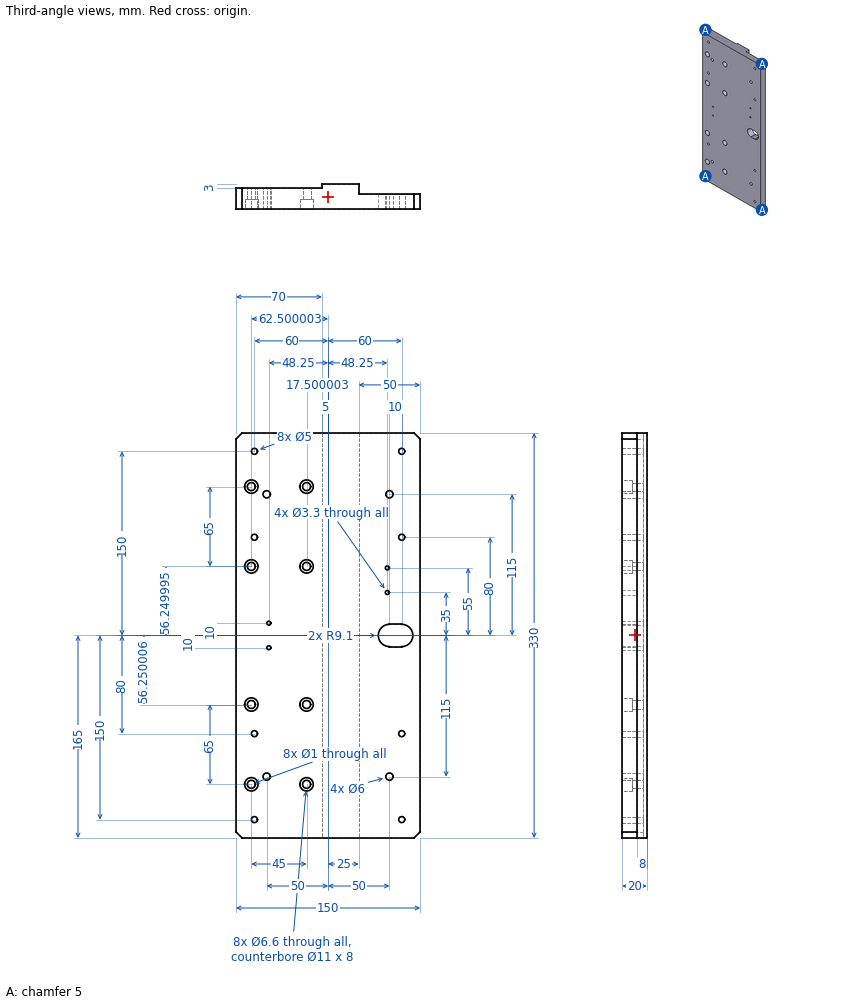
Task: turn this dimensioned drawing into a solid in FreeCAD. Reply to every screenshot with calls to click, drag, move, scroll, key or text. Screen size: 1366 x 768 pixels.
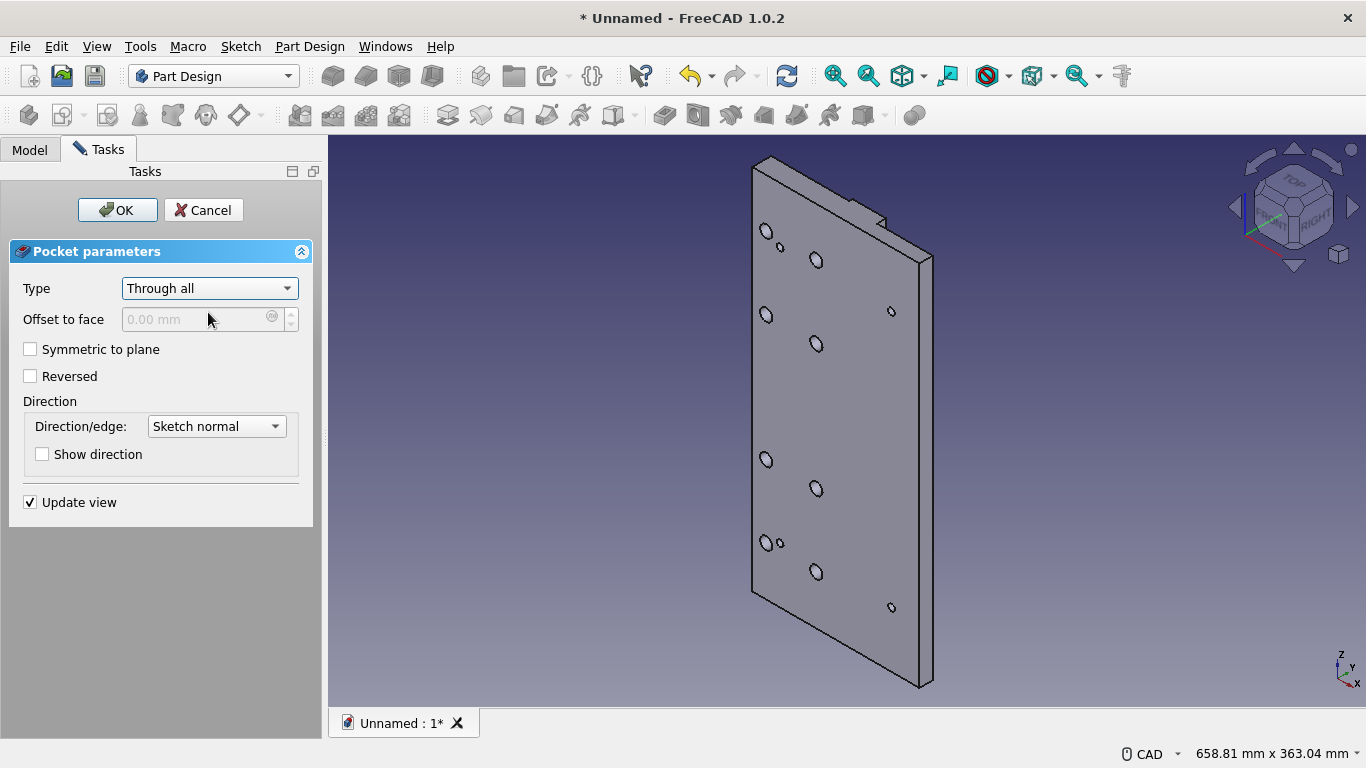
click(118, 210)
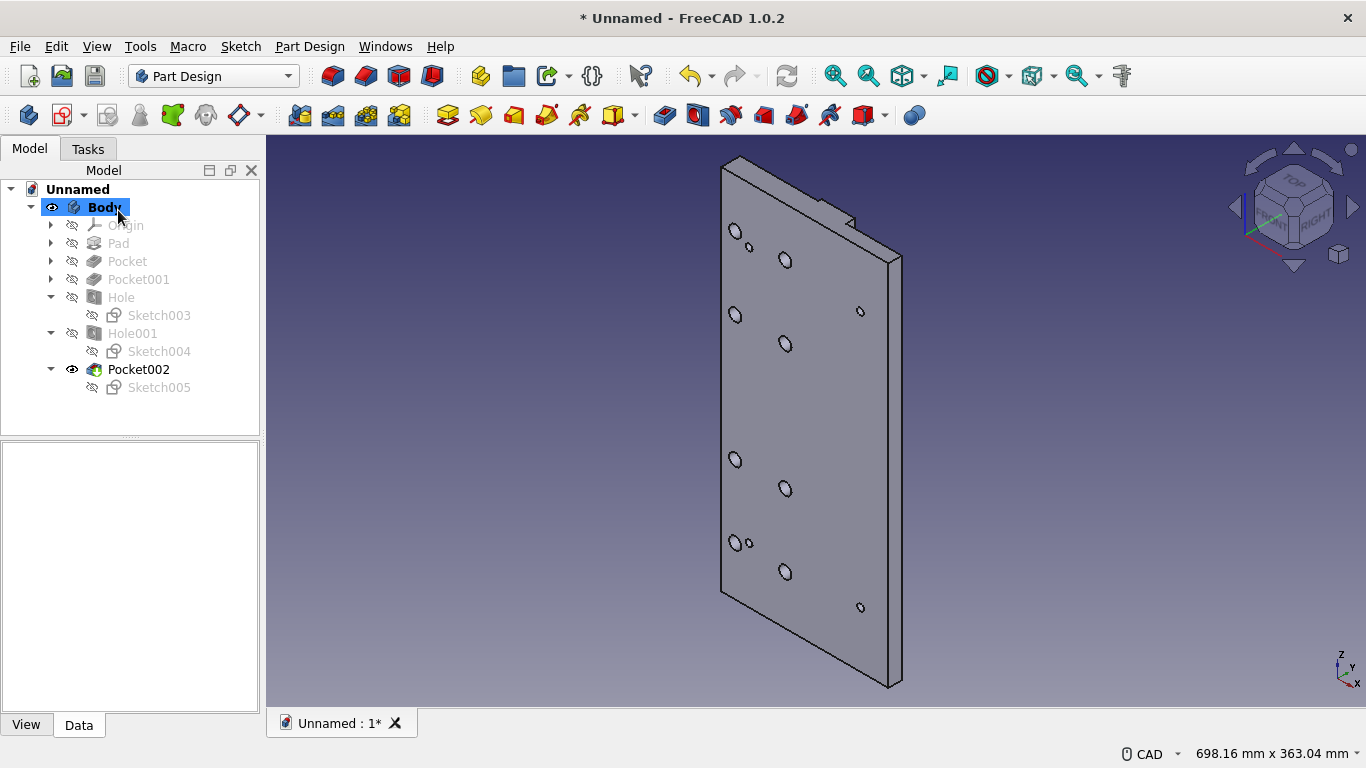
click(829, 440)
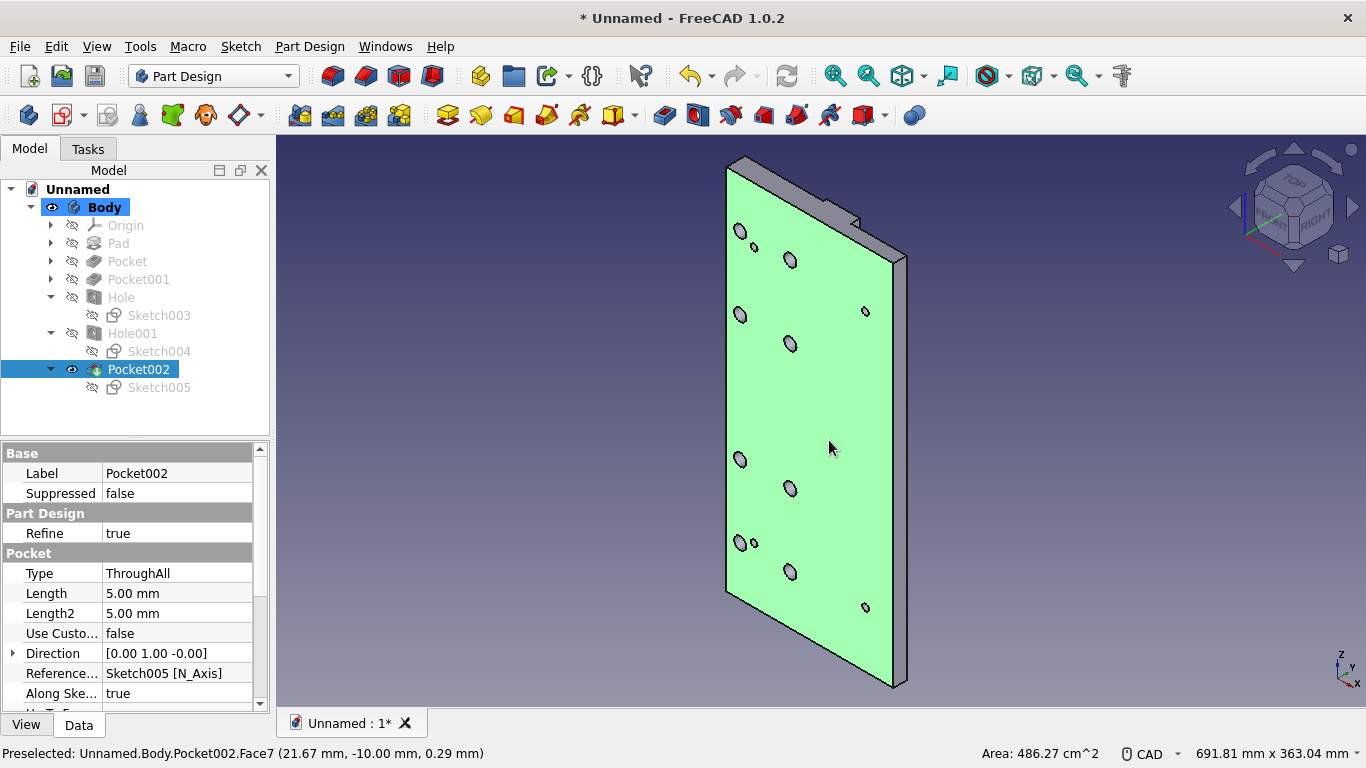
click(62, 116)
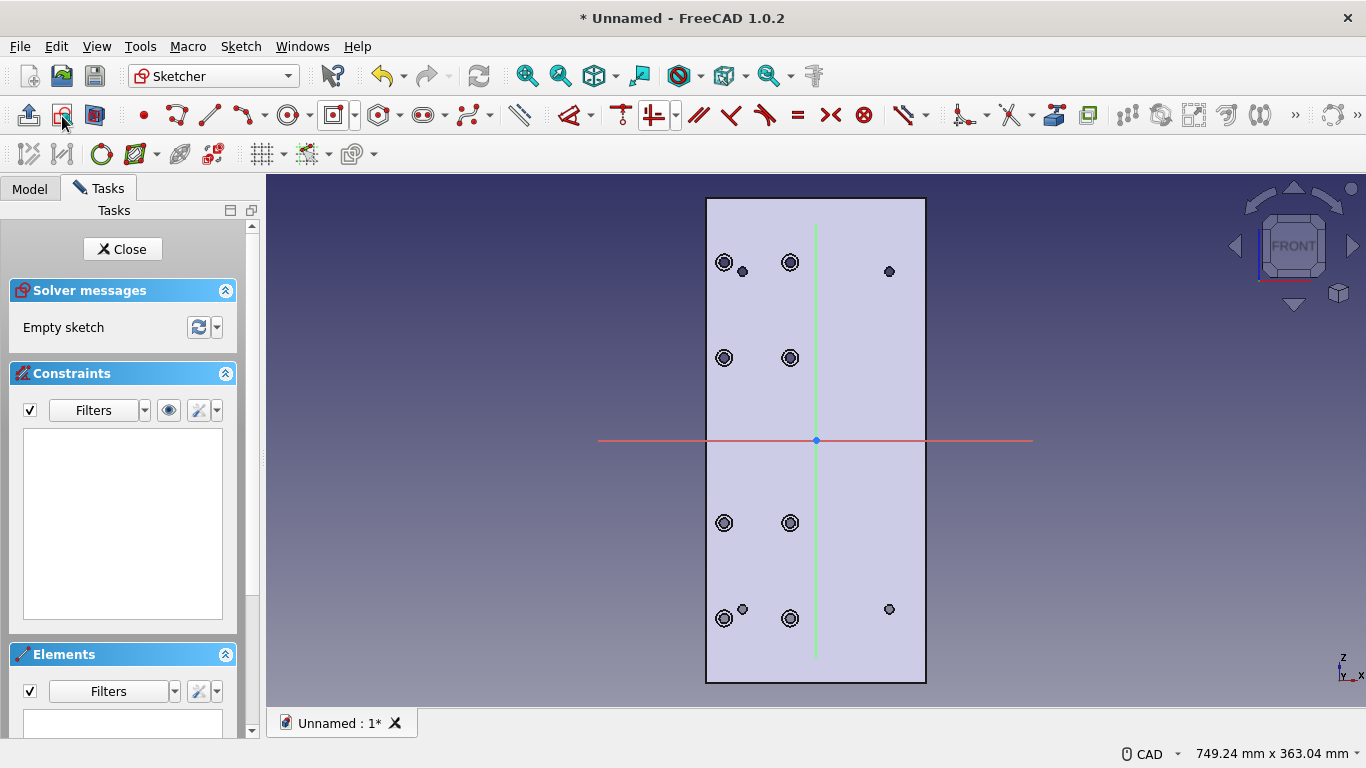
scroll(438, 440, down, 1)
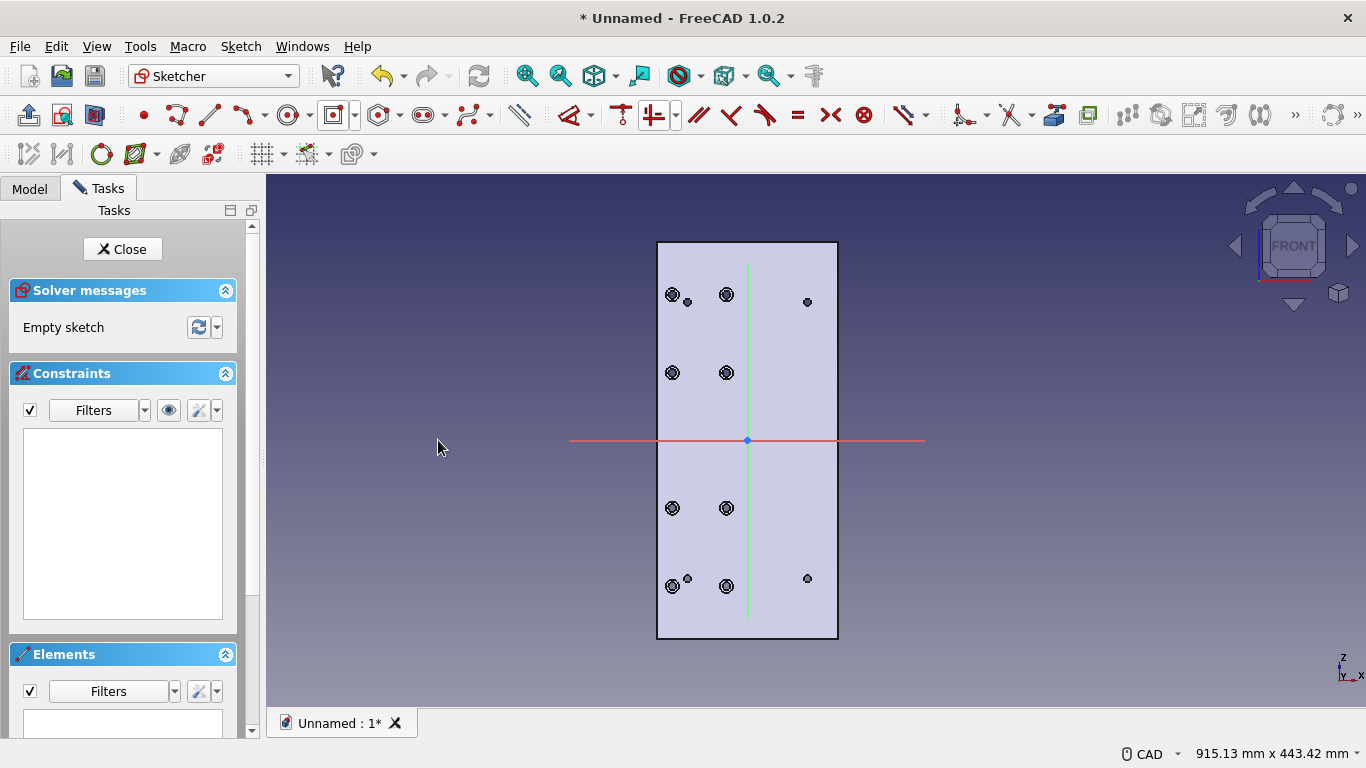
click(288, 116)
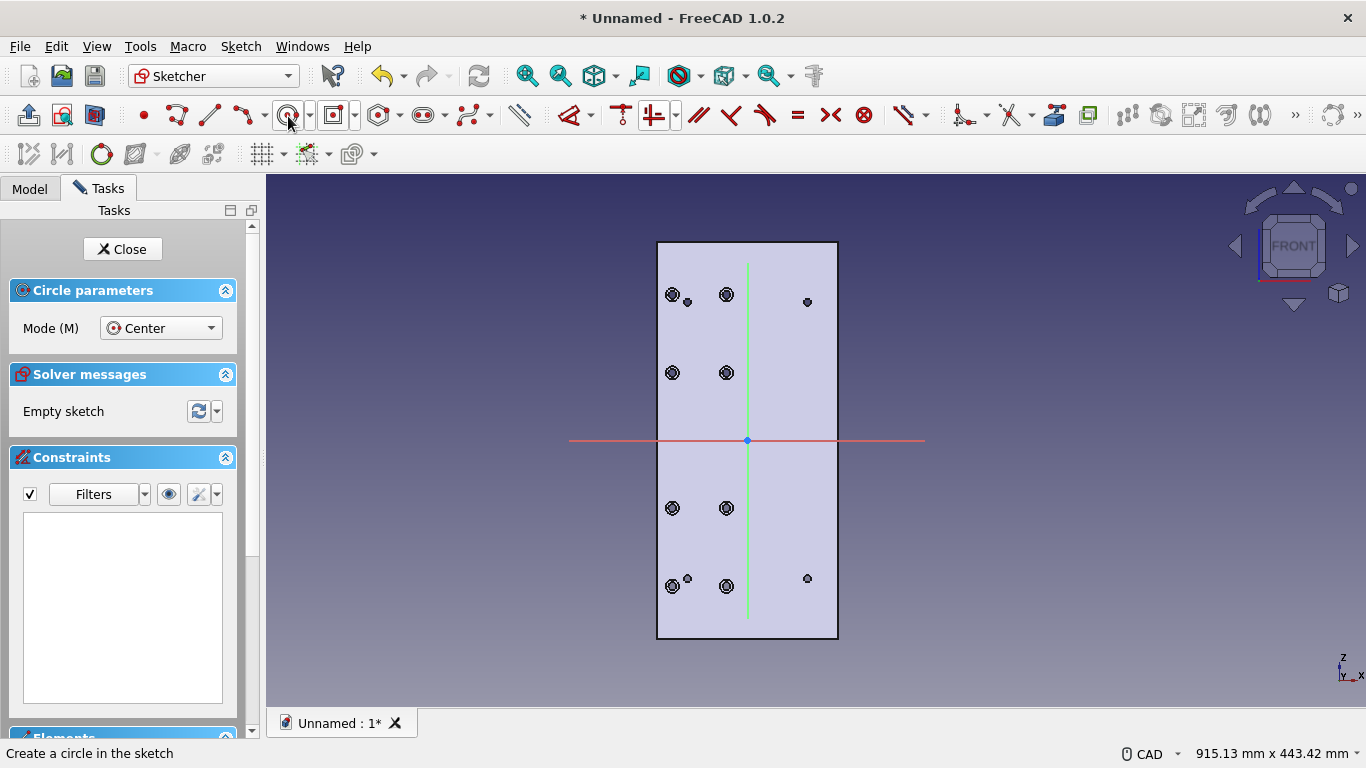
scroll(675, 260, up, 11)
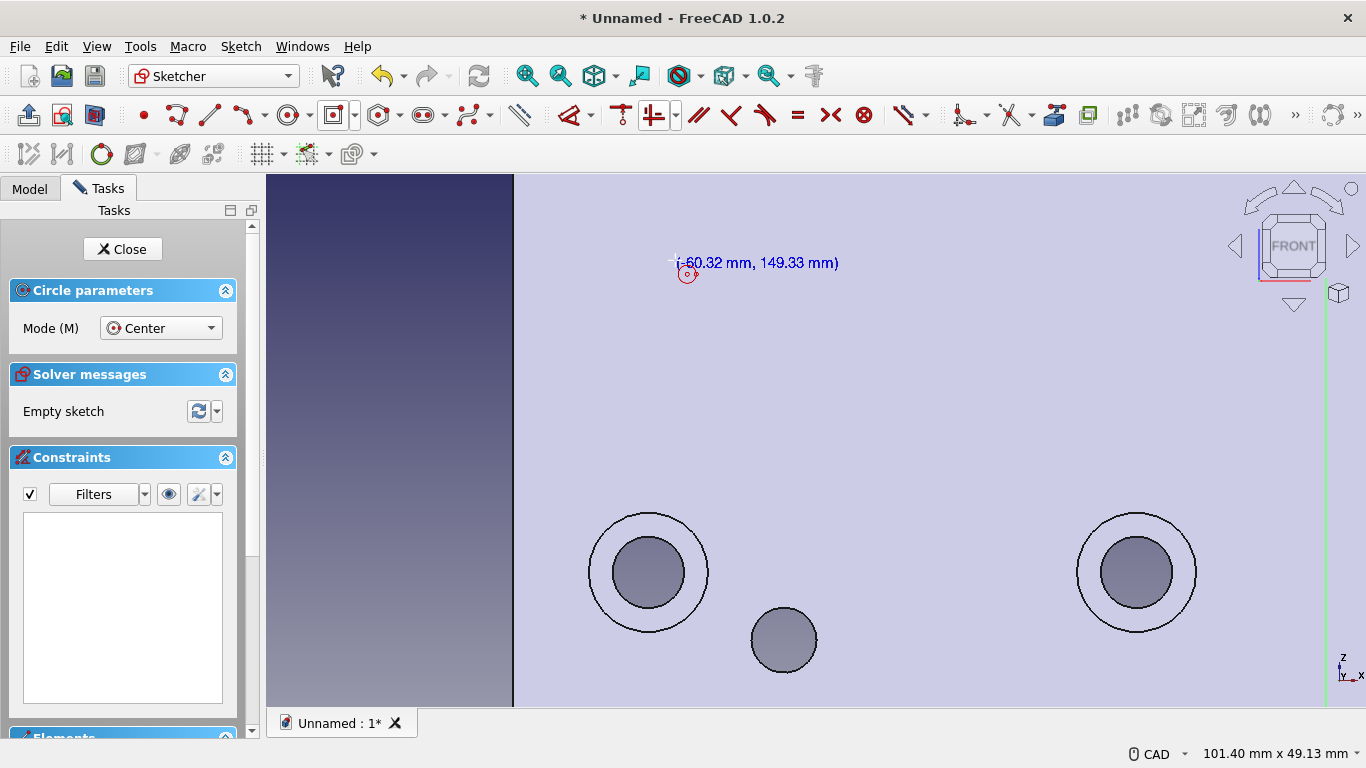
scroll(675, 260, down, 11)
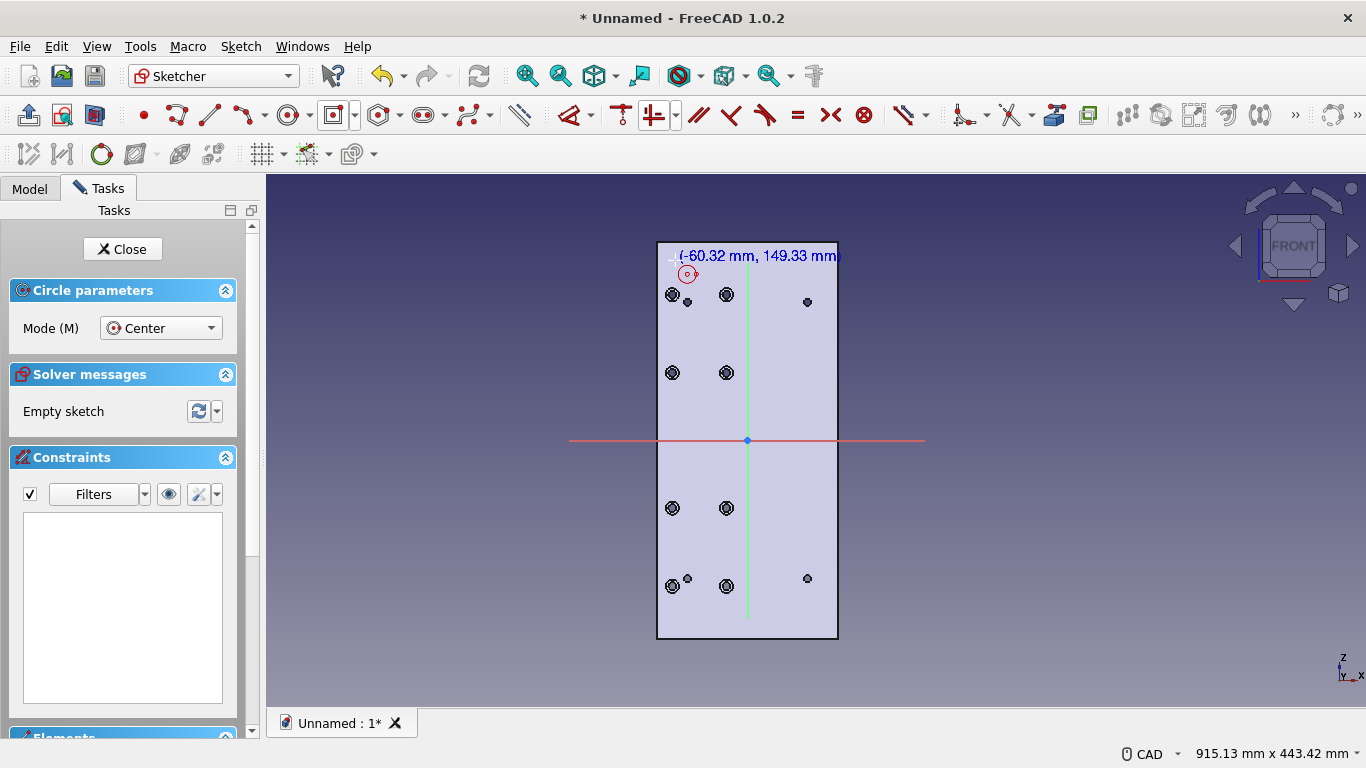
click(675, 260)
move(678, 258)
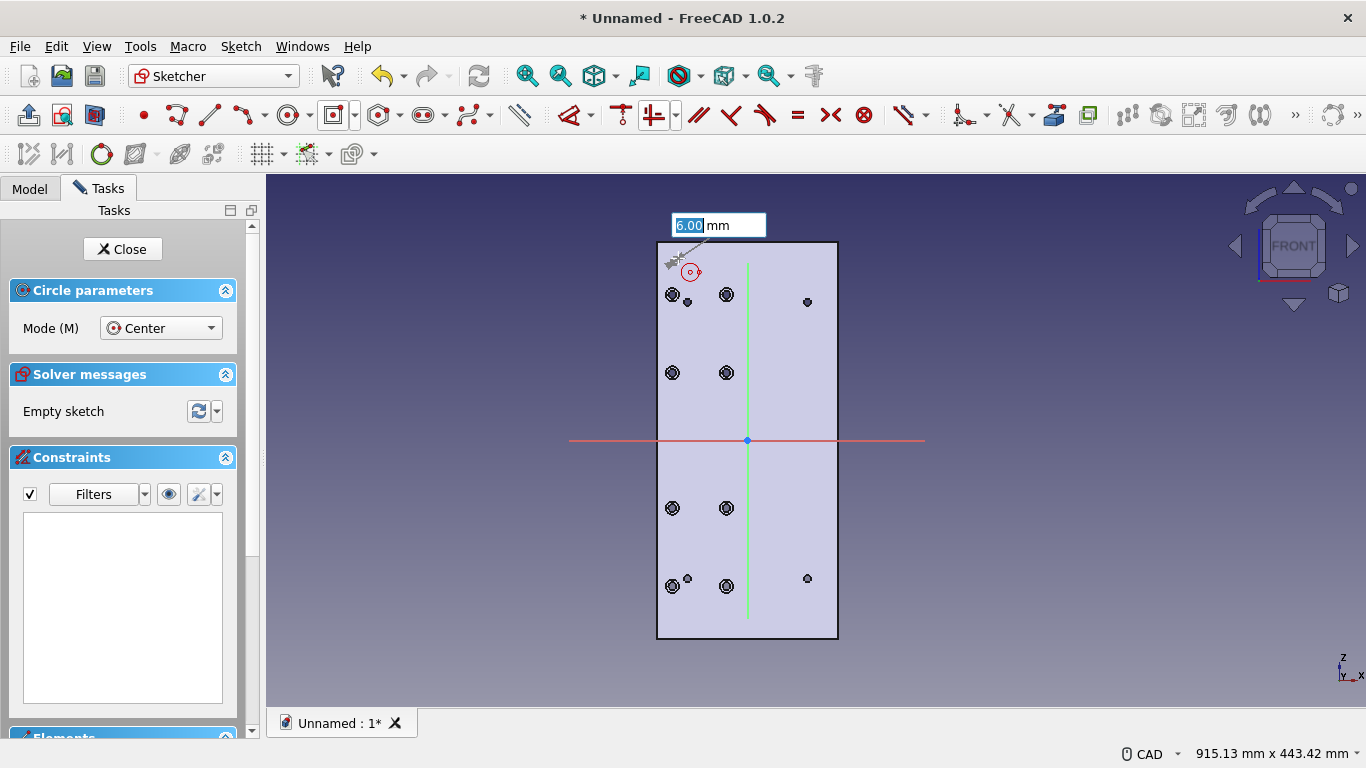
text(5)
key(Return)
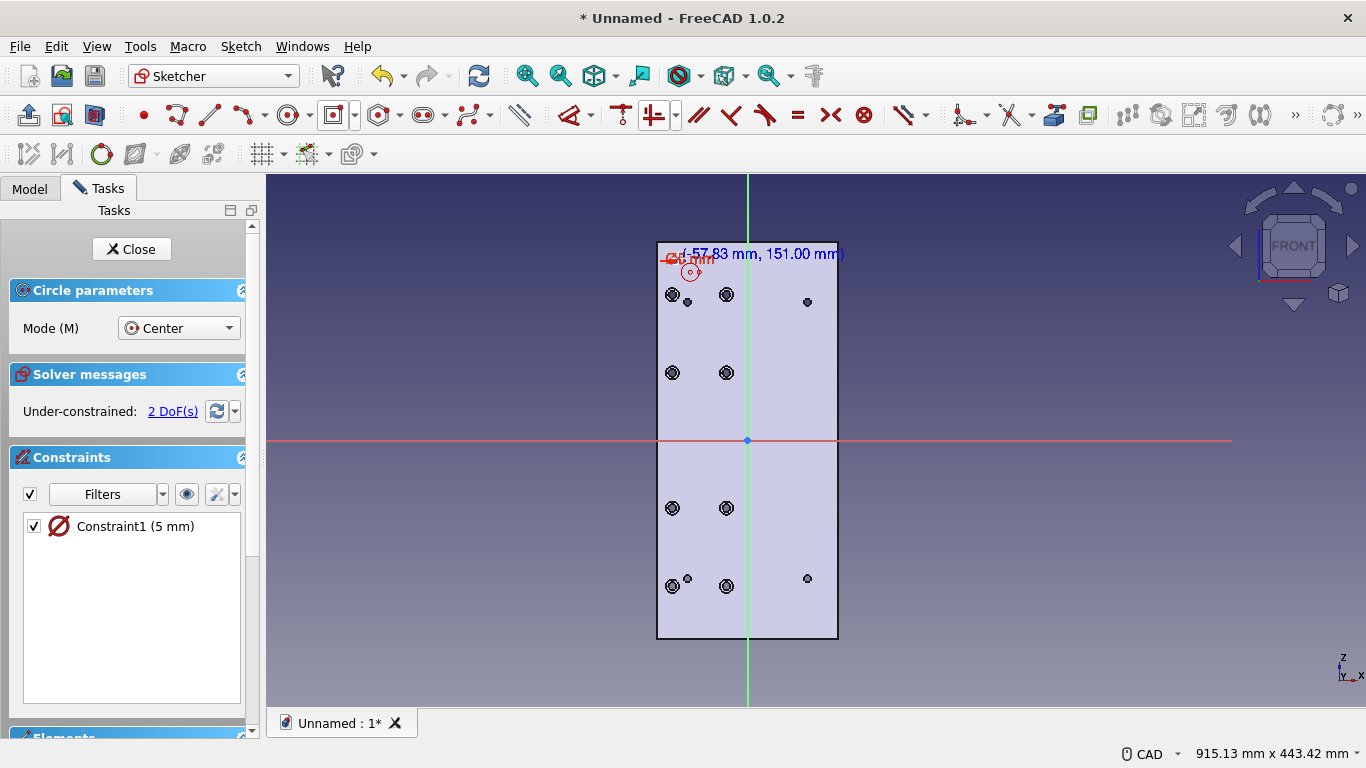
scroll(820, 260, up, 11)